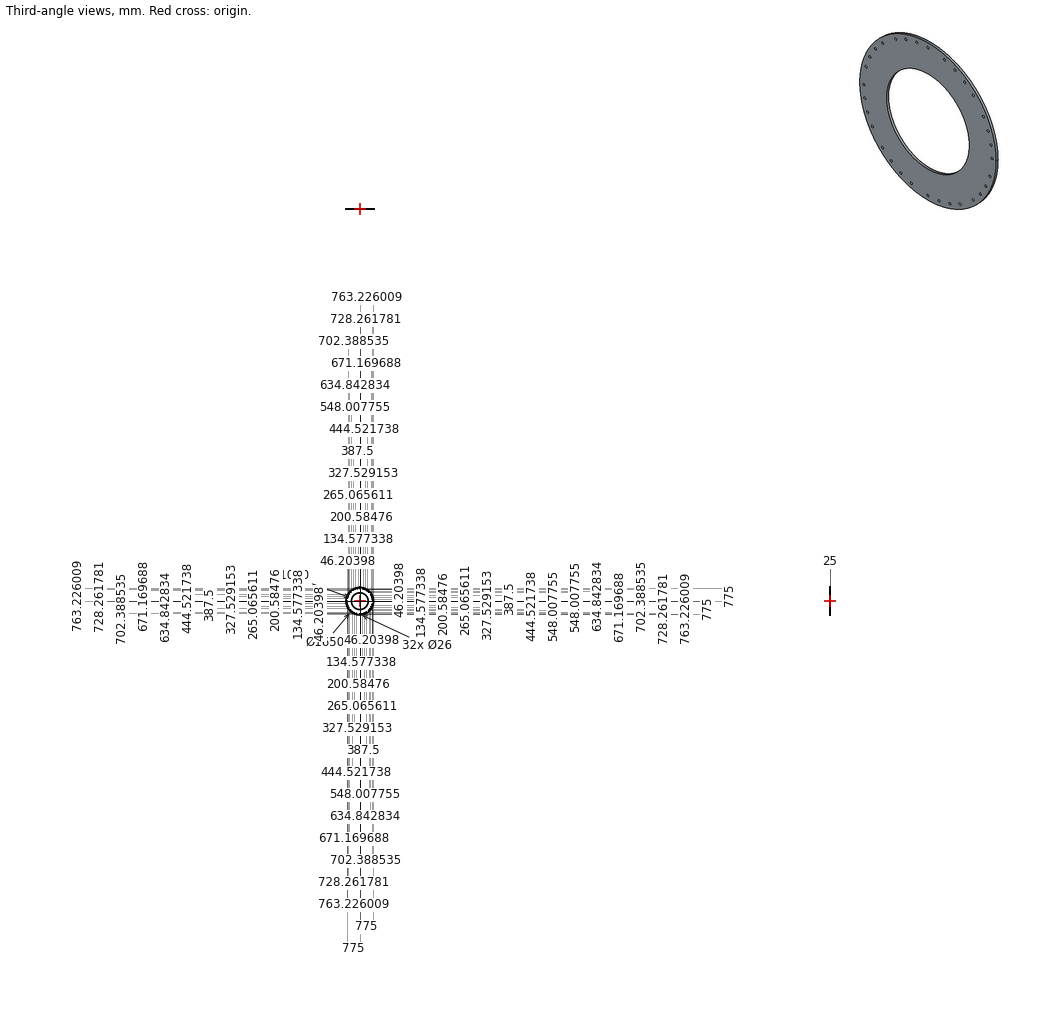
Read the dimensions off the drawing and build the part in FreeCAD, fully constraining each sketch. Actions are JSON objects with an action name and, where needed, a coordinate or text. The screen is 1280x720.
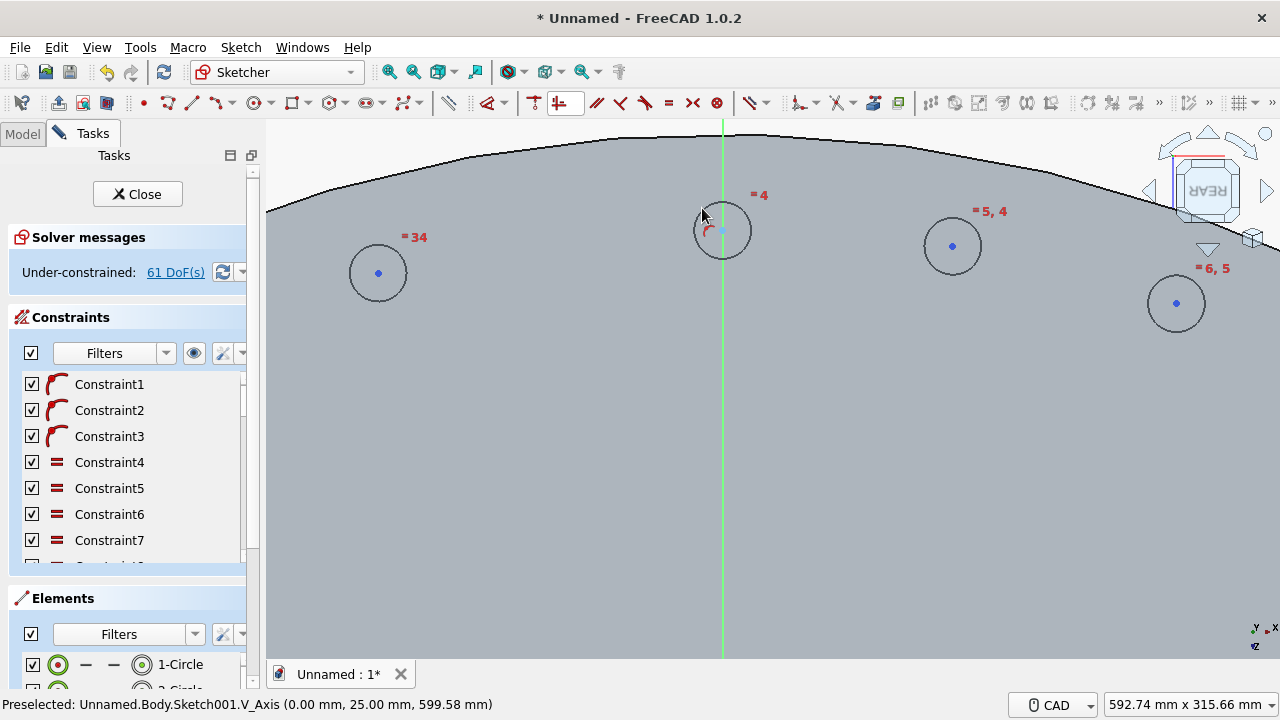
{"action": "left_click", "coordinate": [703, 210]}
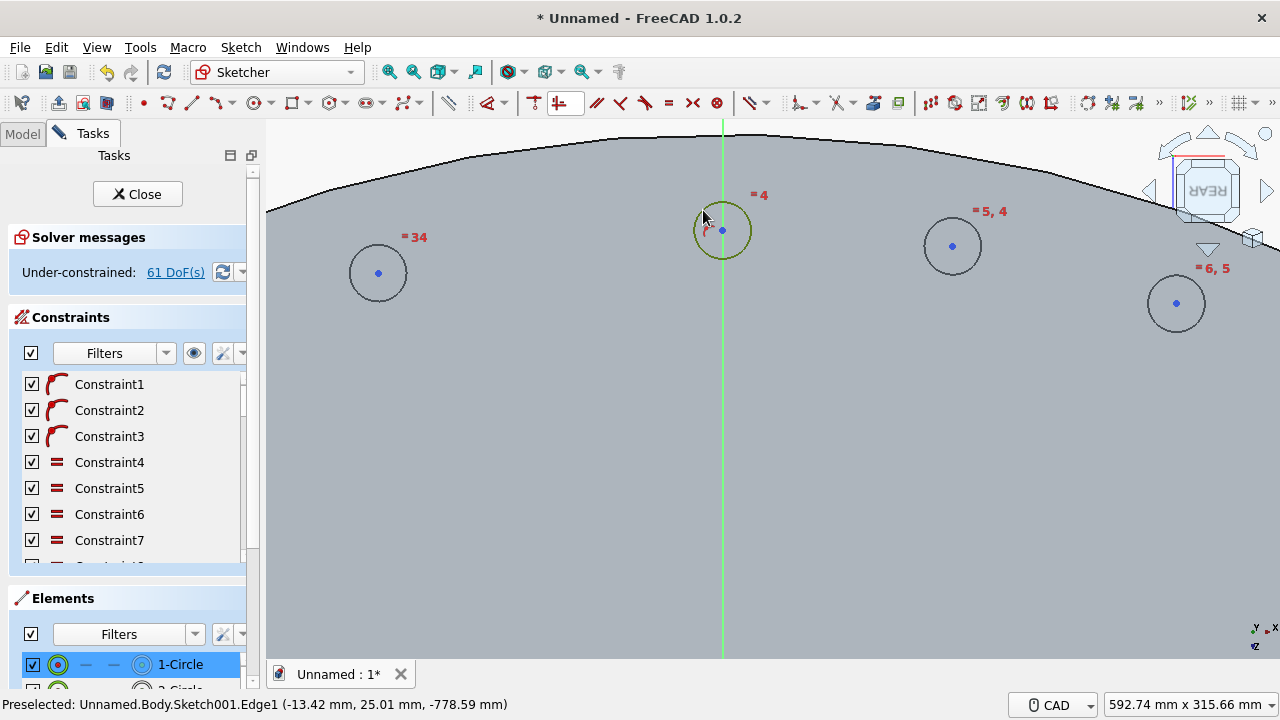
{"action": "key", "text": "k o"}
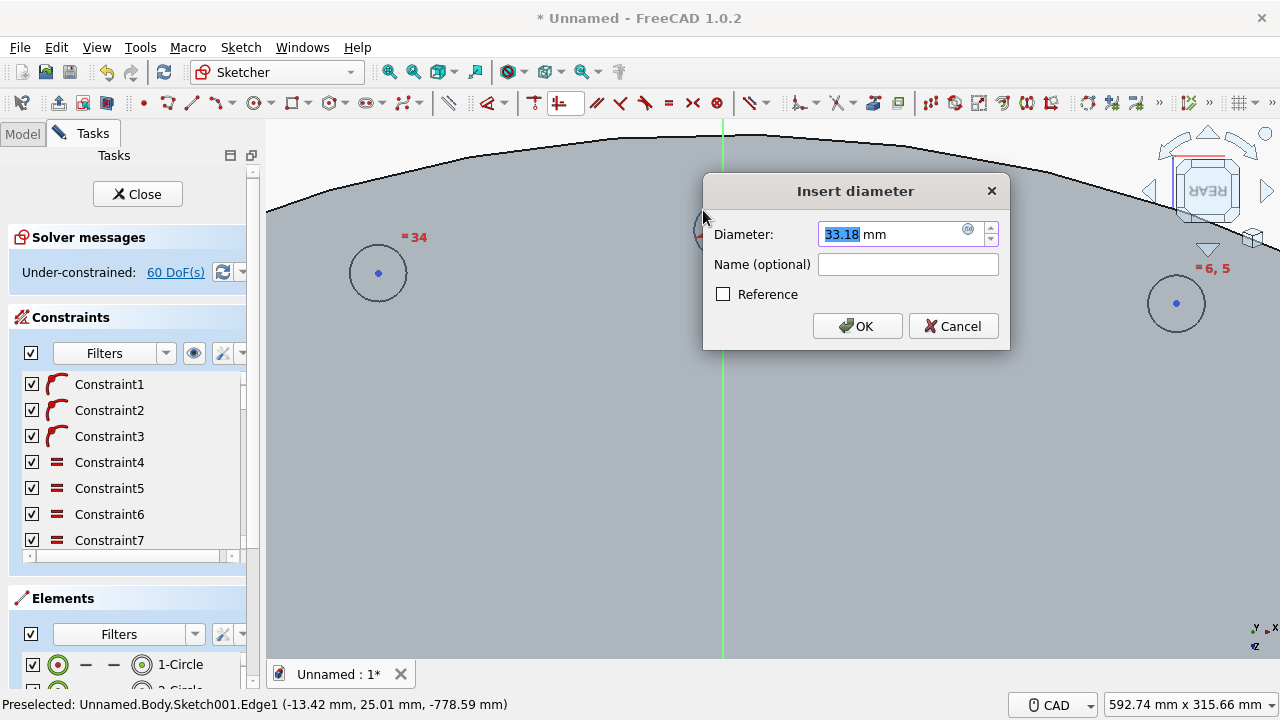
{"action": "type", "text": "26"}
{"action": "key", "text": "Return"}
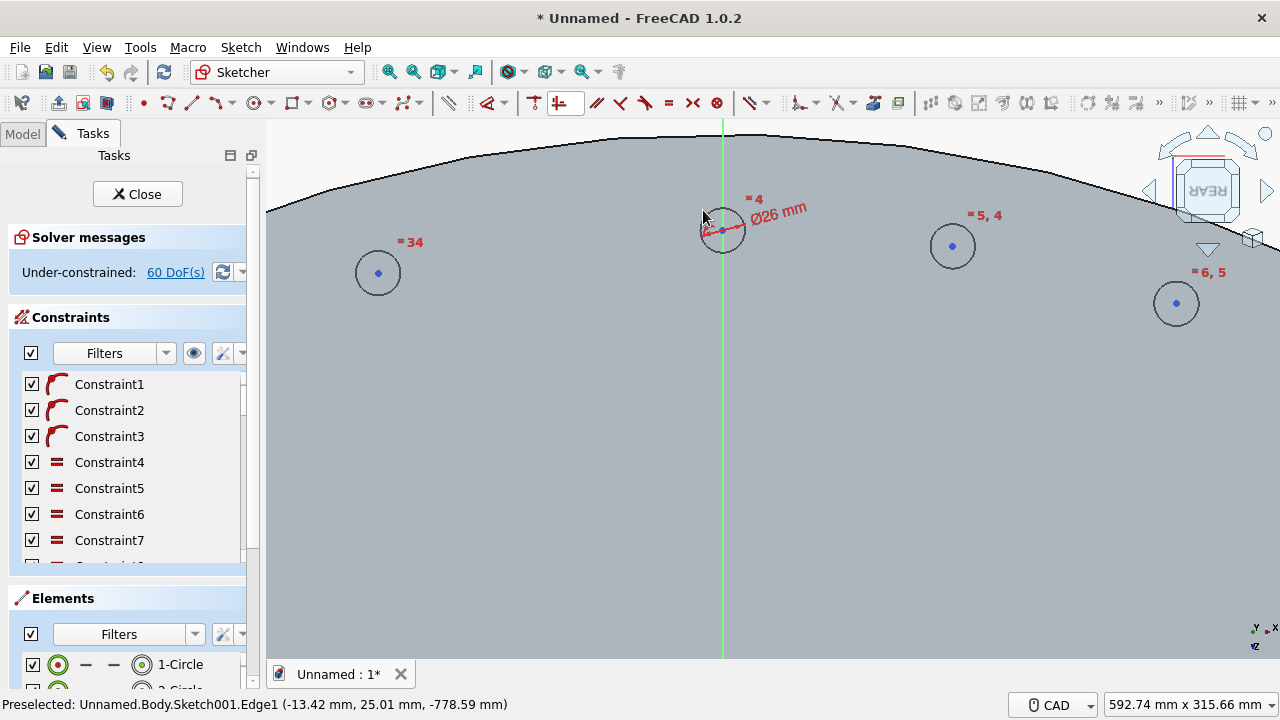
{"action": "scroll", "coordinate": [702, 208], "scroll_direction": "down", "scroll_amount": 10}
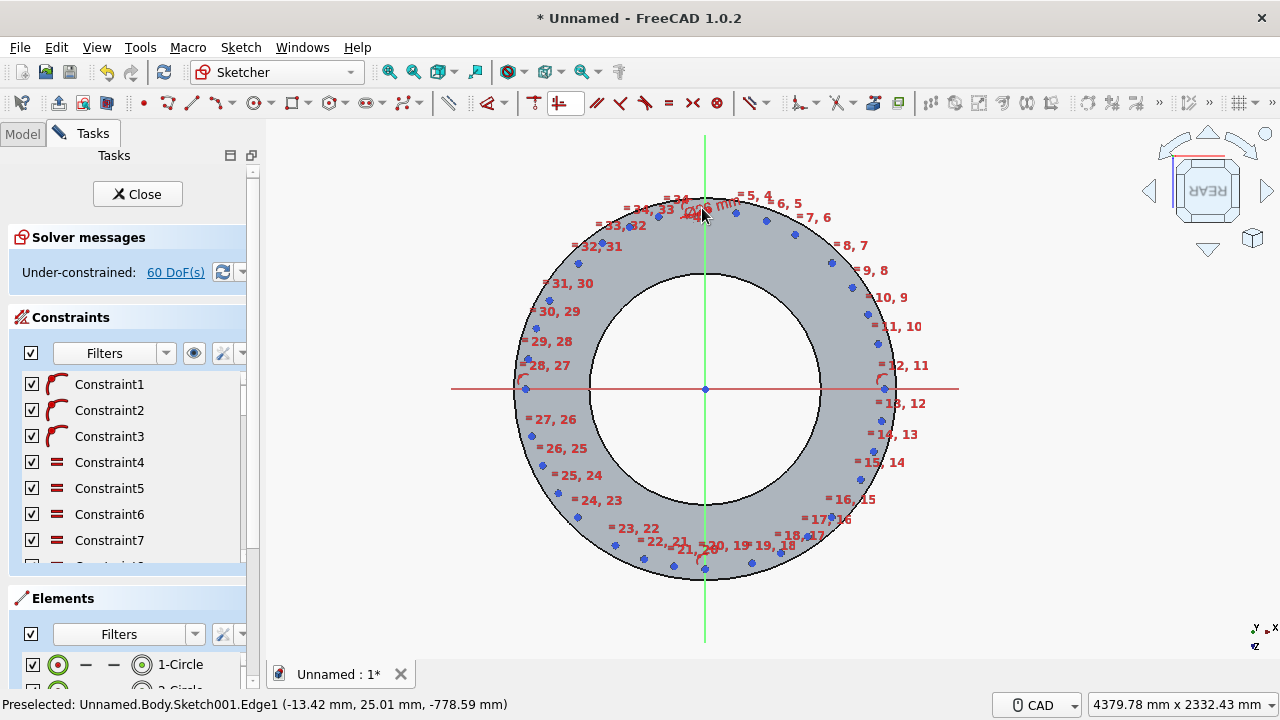
{"action": "left_click", "coordinate": [705, 211]}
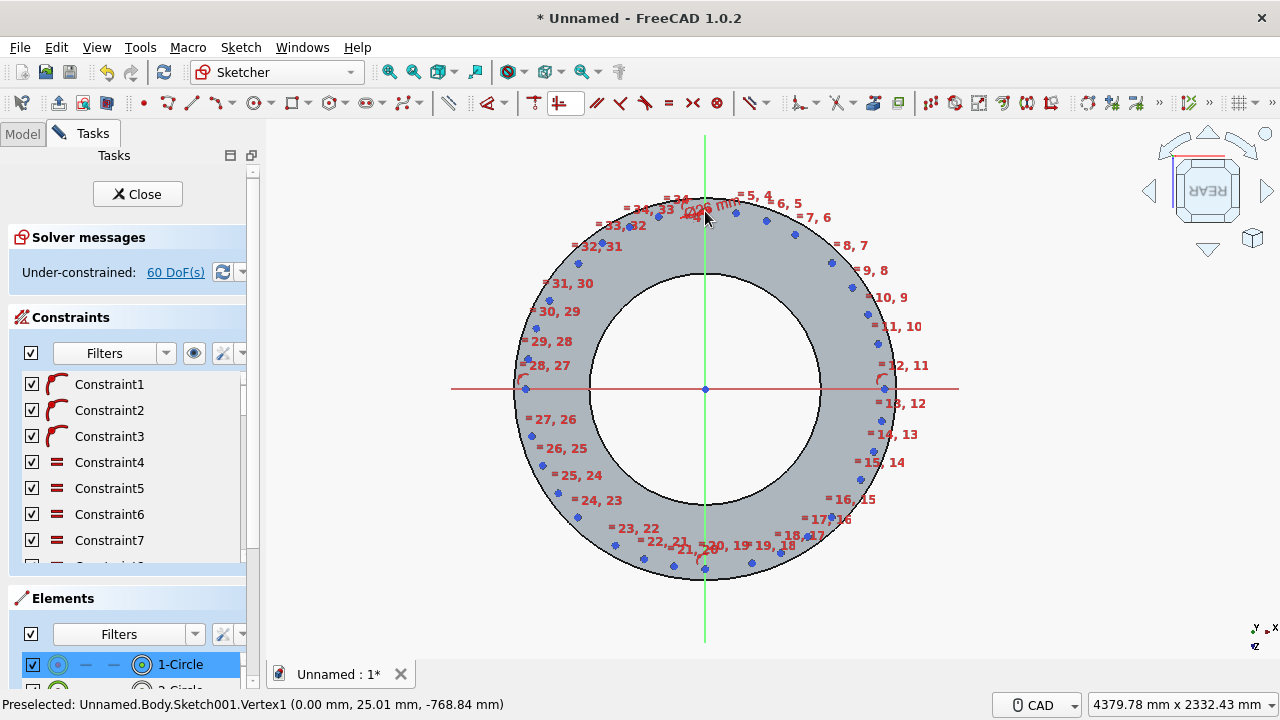
{"action": "key", "text": "i"}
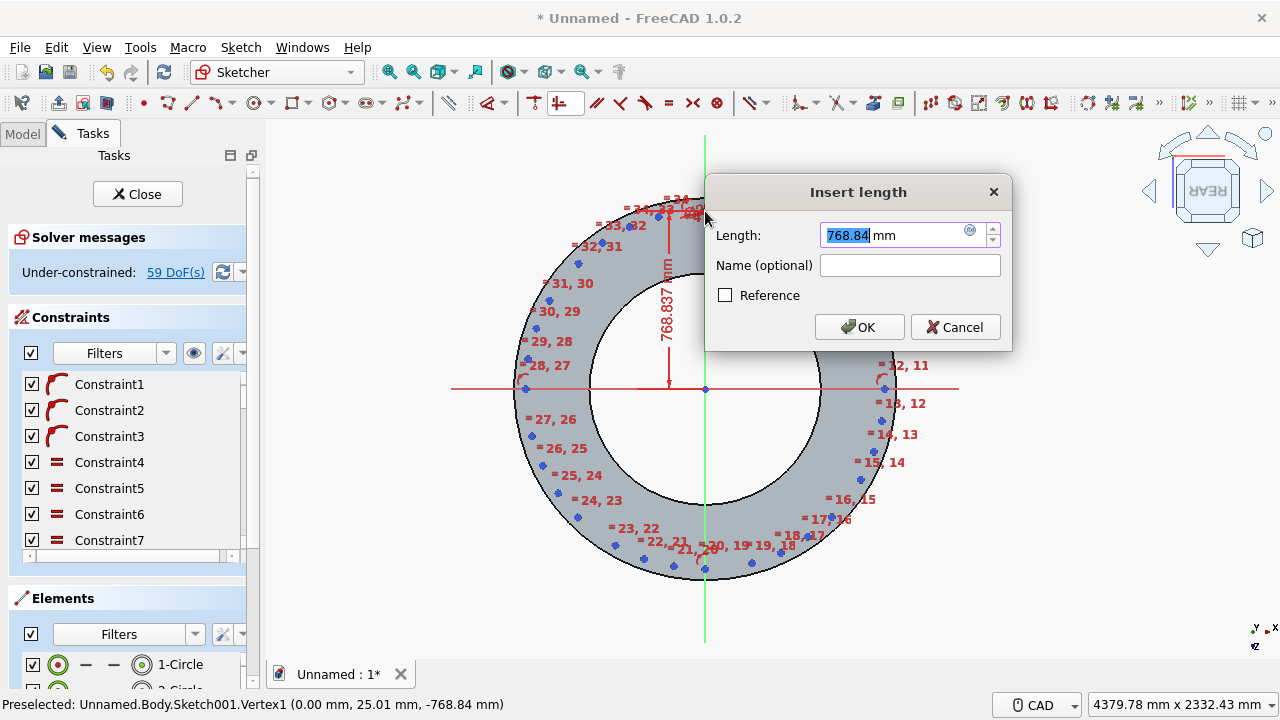
{"action": "type", "text": "775"}
{"action": "key", "text": "Return"}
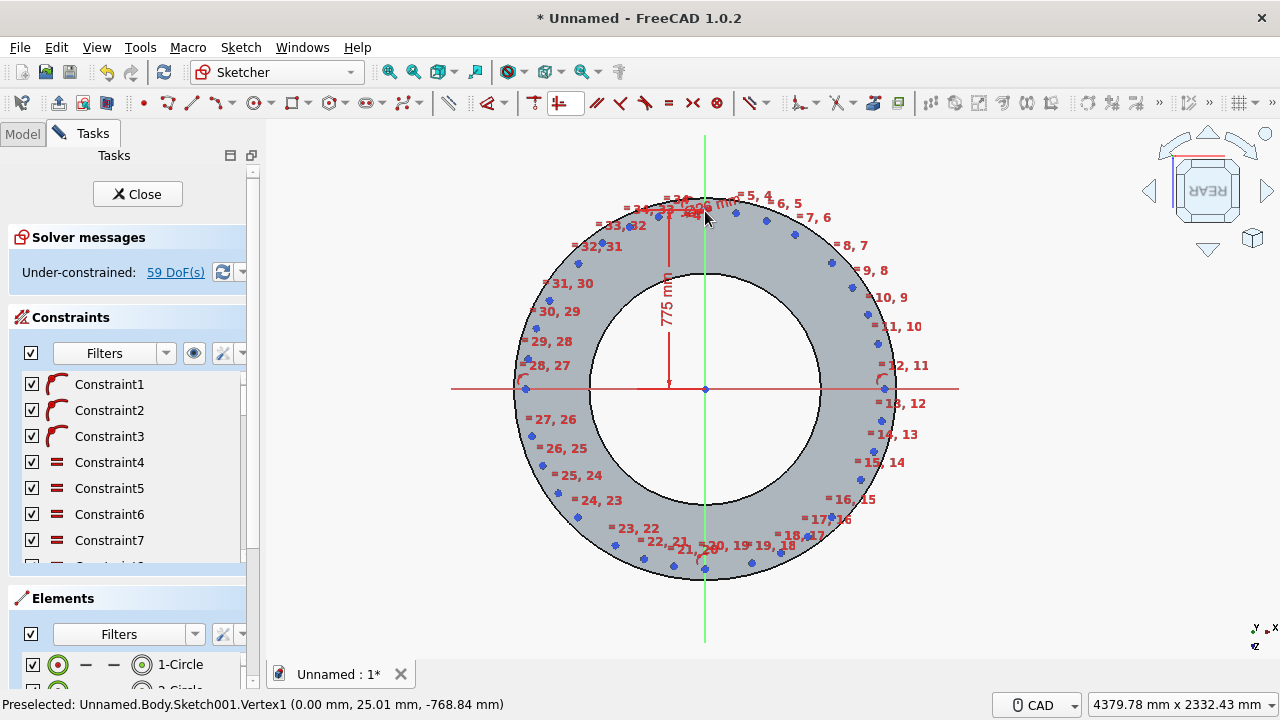
{"action": "left_click", "coordinate": [885, 389]}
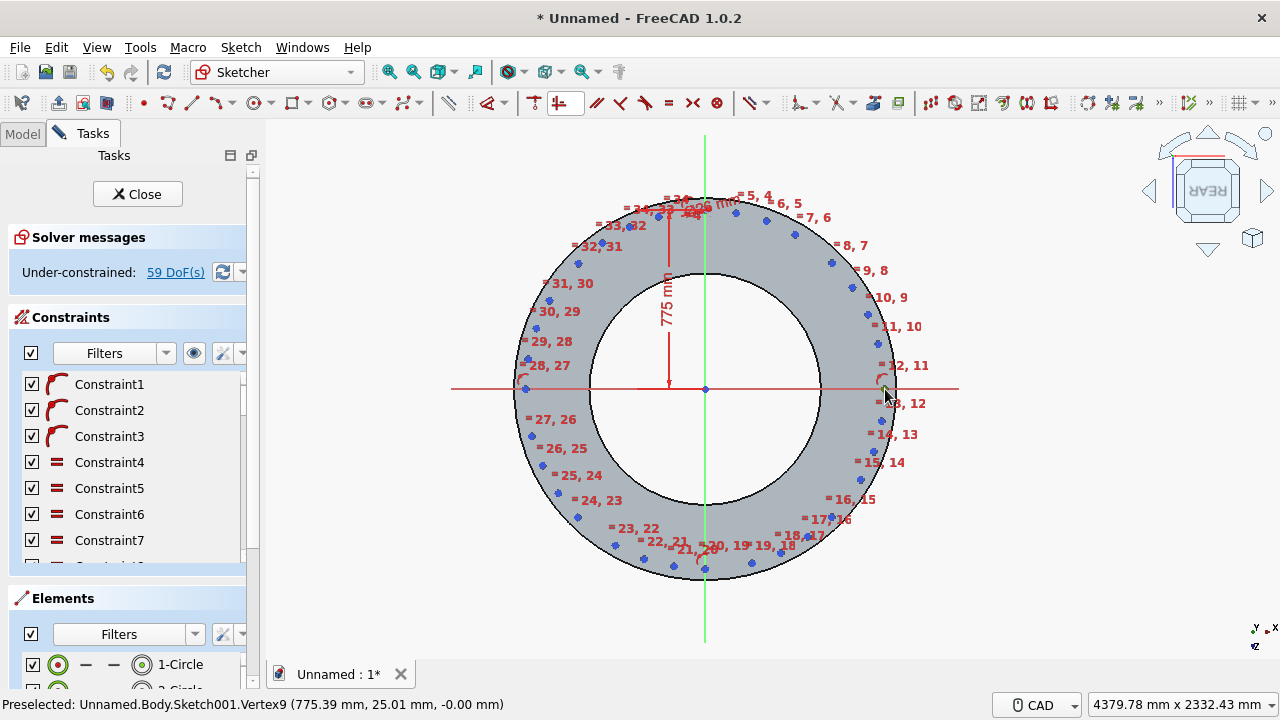
{"action": "key", "text": "l"}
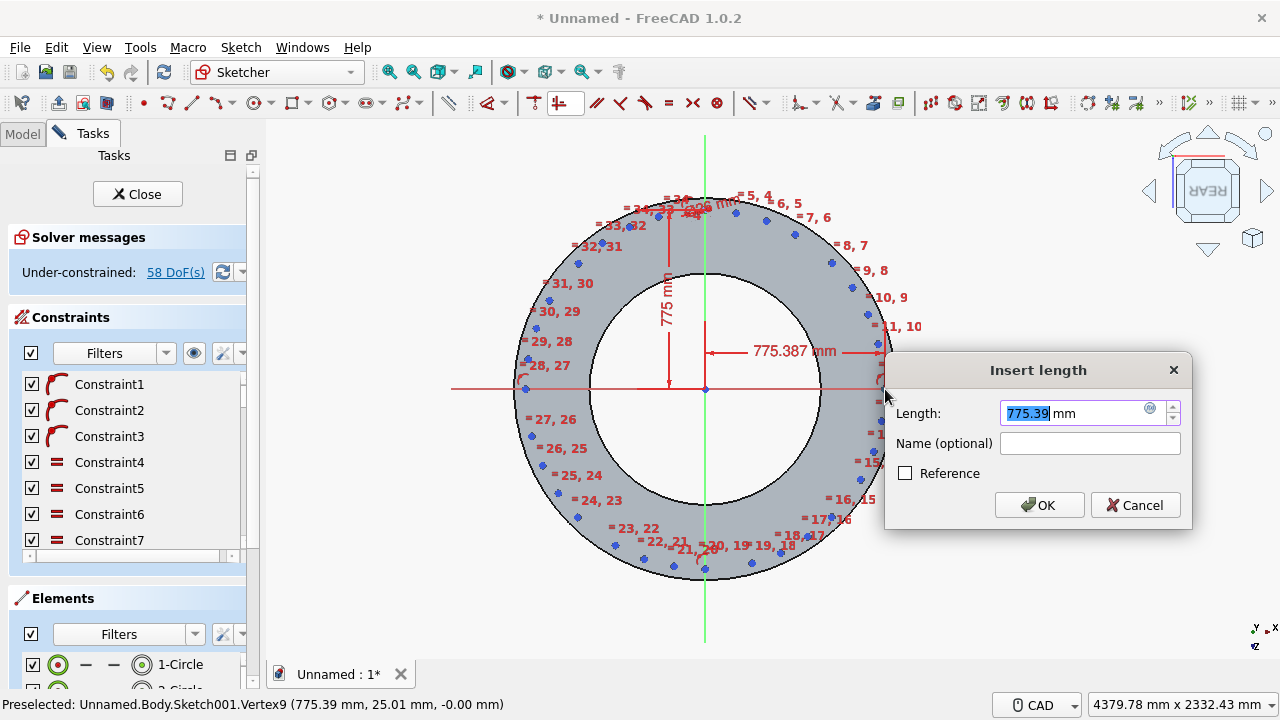
{"action": "type", "text": "775"}
{"action": "key", "text": "Return"}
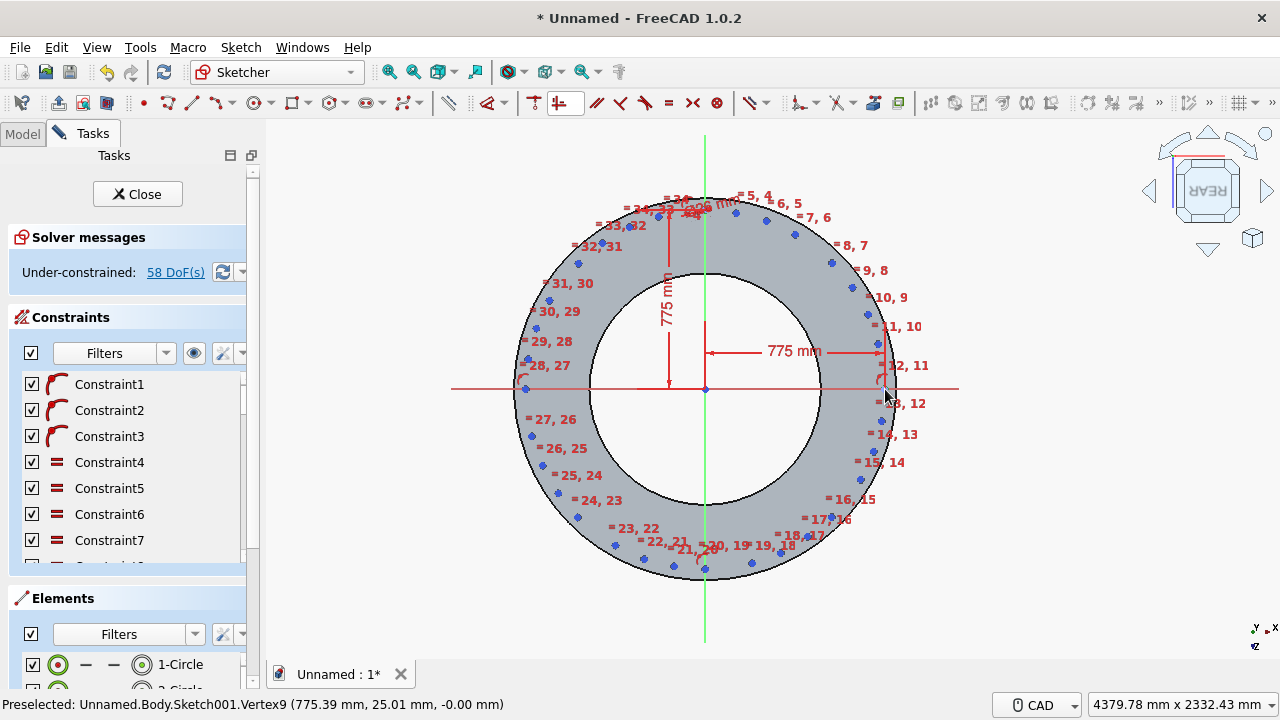
{"action": "left_click", "coordinate": [705, 569]}